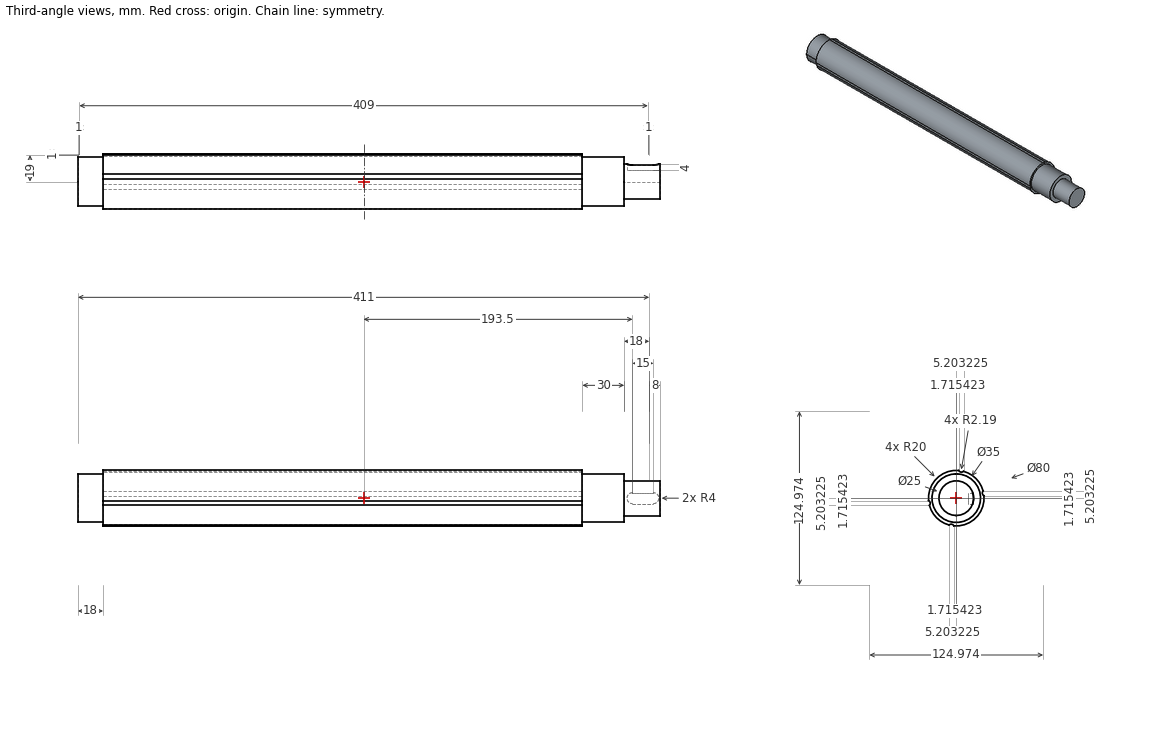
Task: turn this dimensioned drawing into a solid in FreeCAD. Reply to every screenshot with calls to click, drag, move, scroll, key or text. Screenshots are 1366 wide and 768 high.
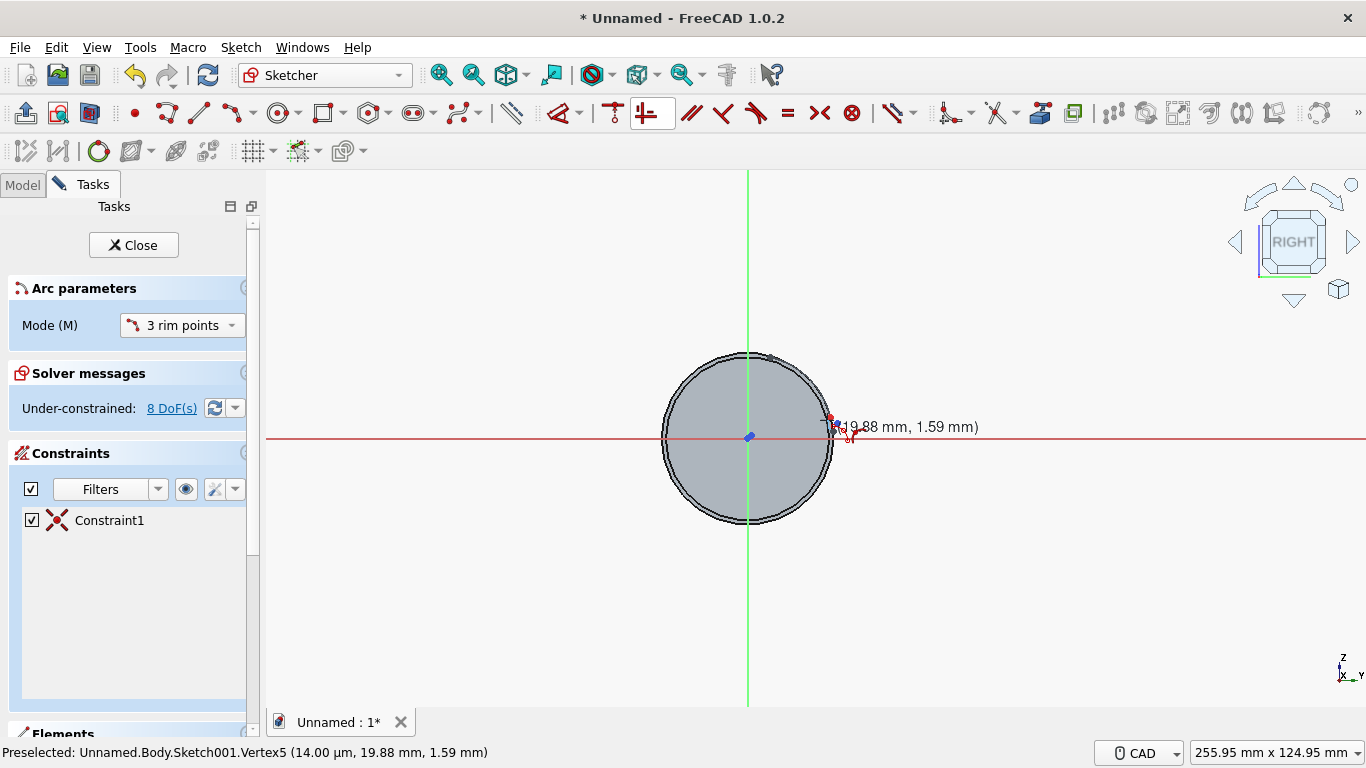
scroll(740, 524, up, 4)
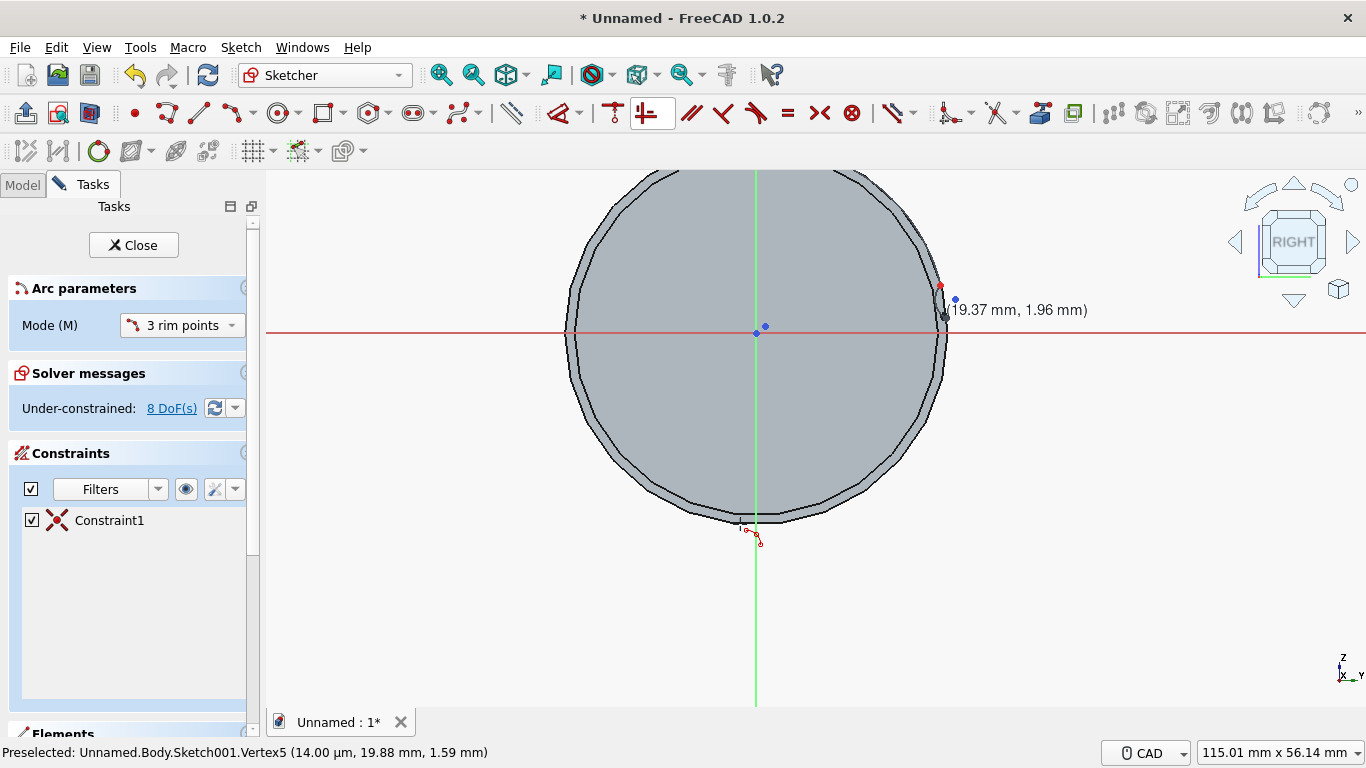
click(740, 524)
click(892, 469)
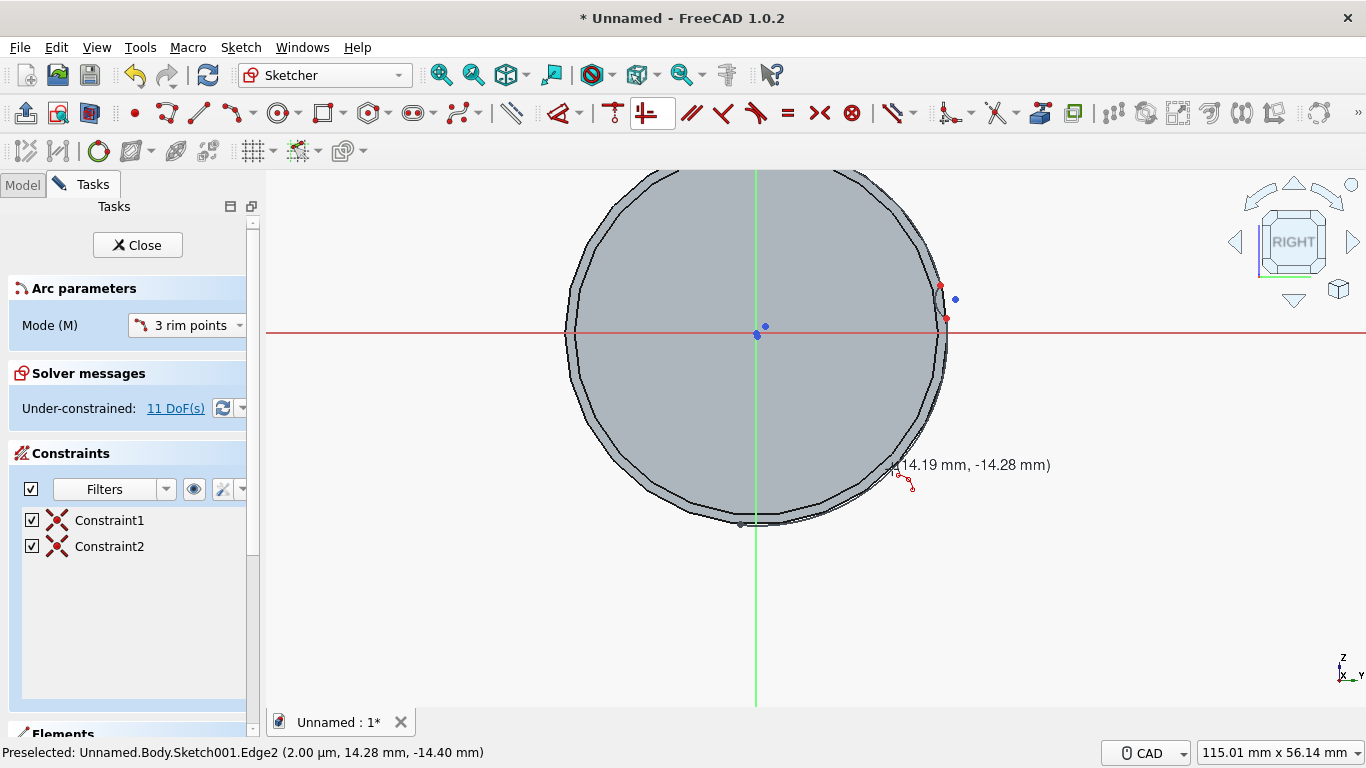
click(740, 525)
click(707, 518)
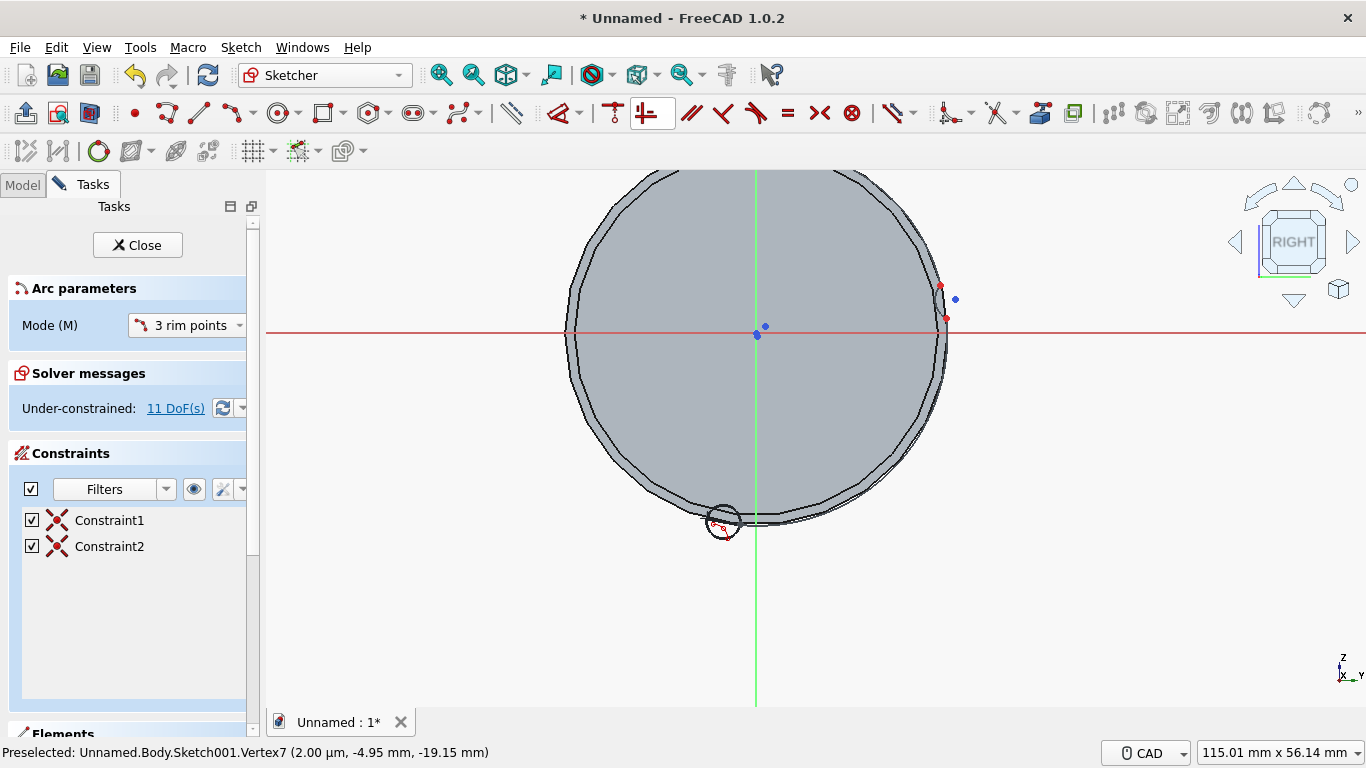
scroll(725, 513, up, 4)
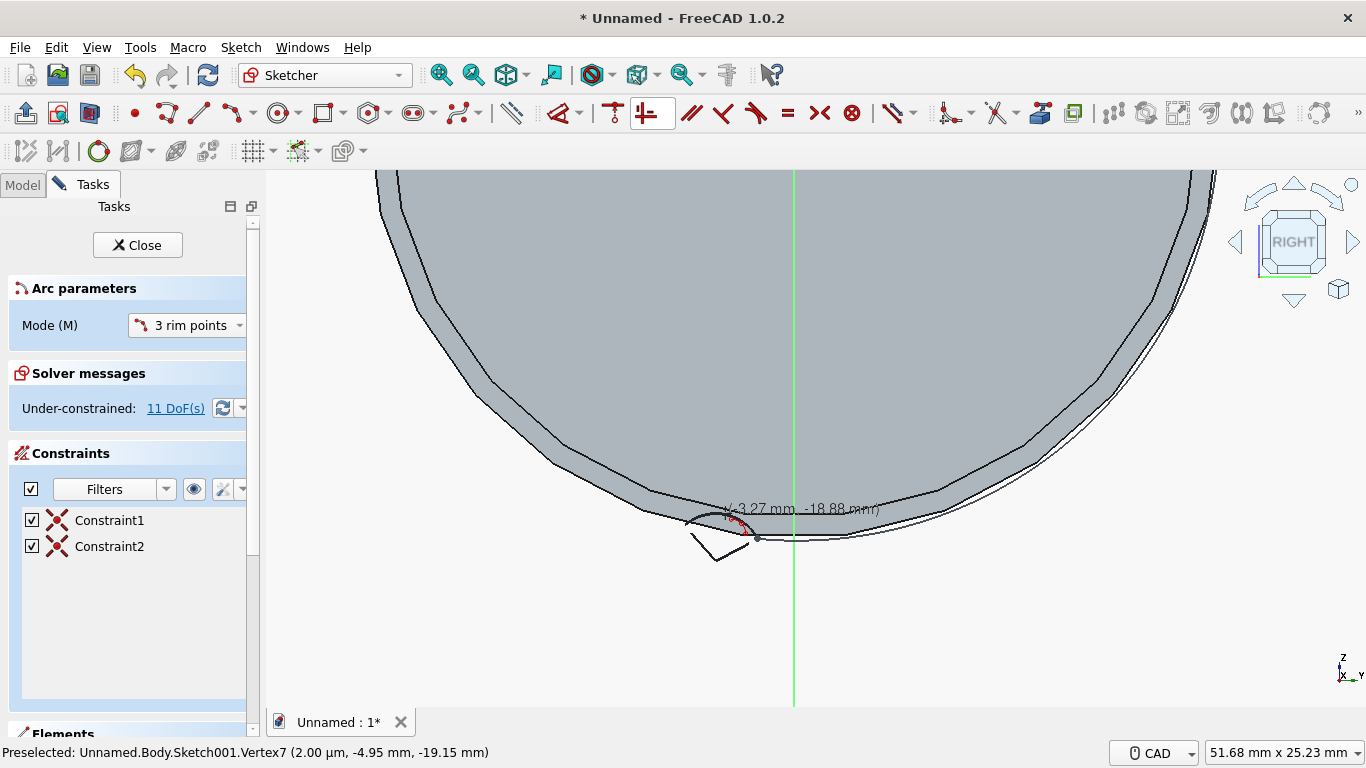
click(724, 511)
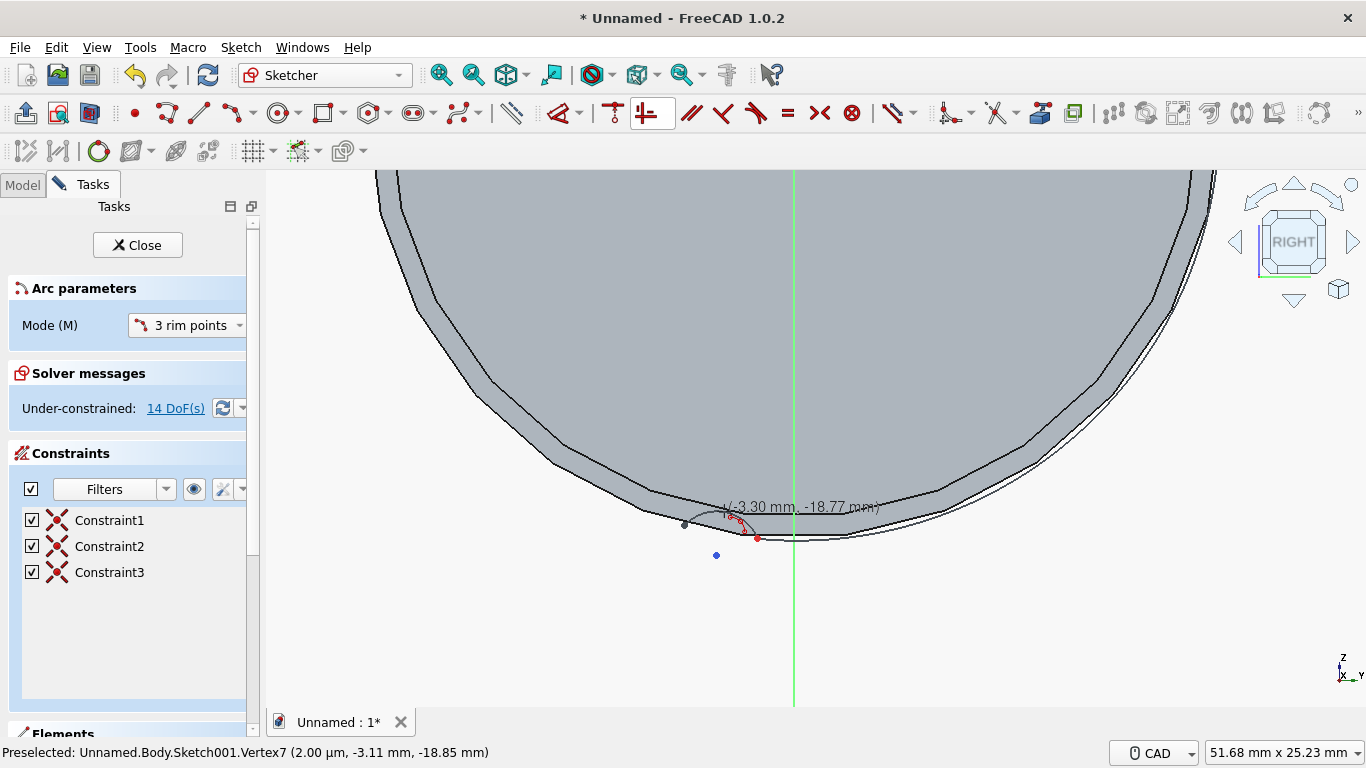
scroll(736, 521, down, 8)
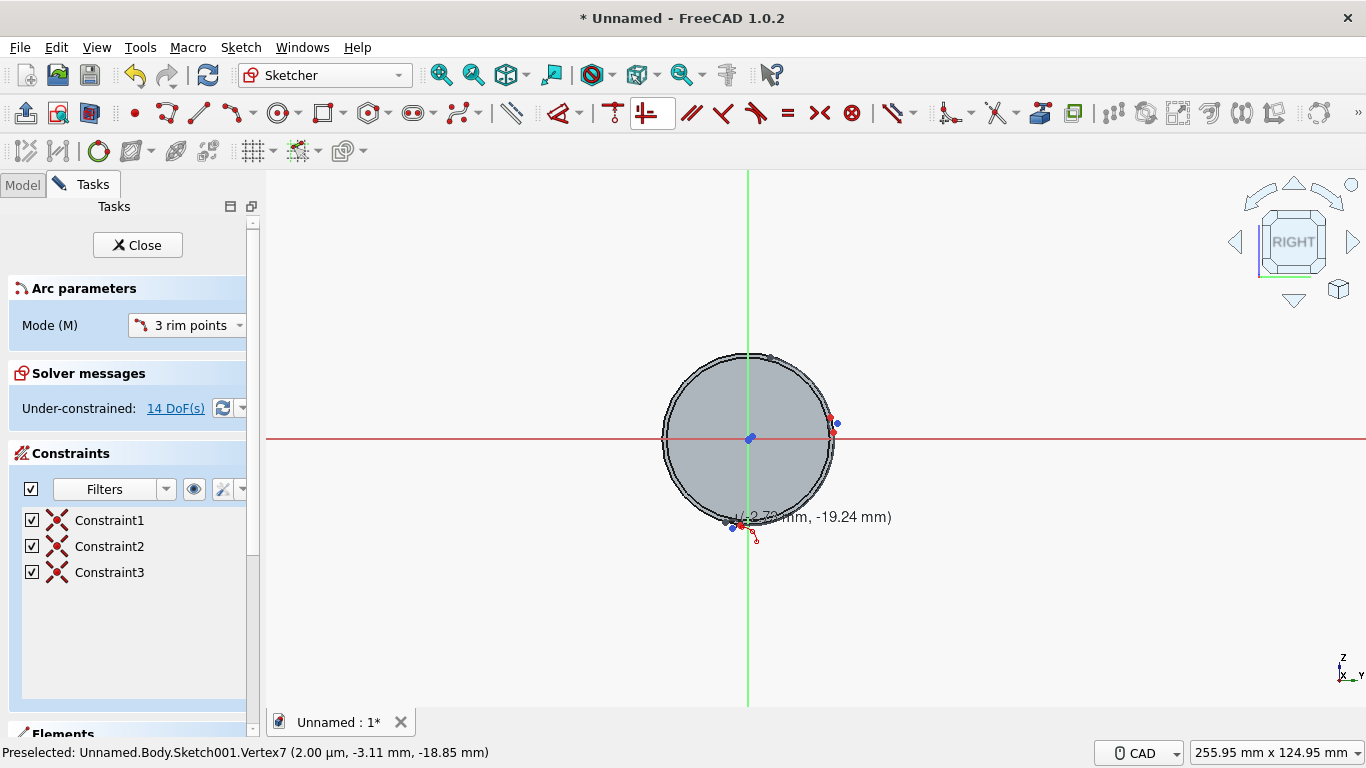
scroll(726, 522, up, 3)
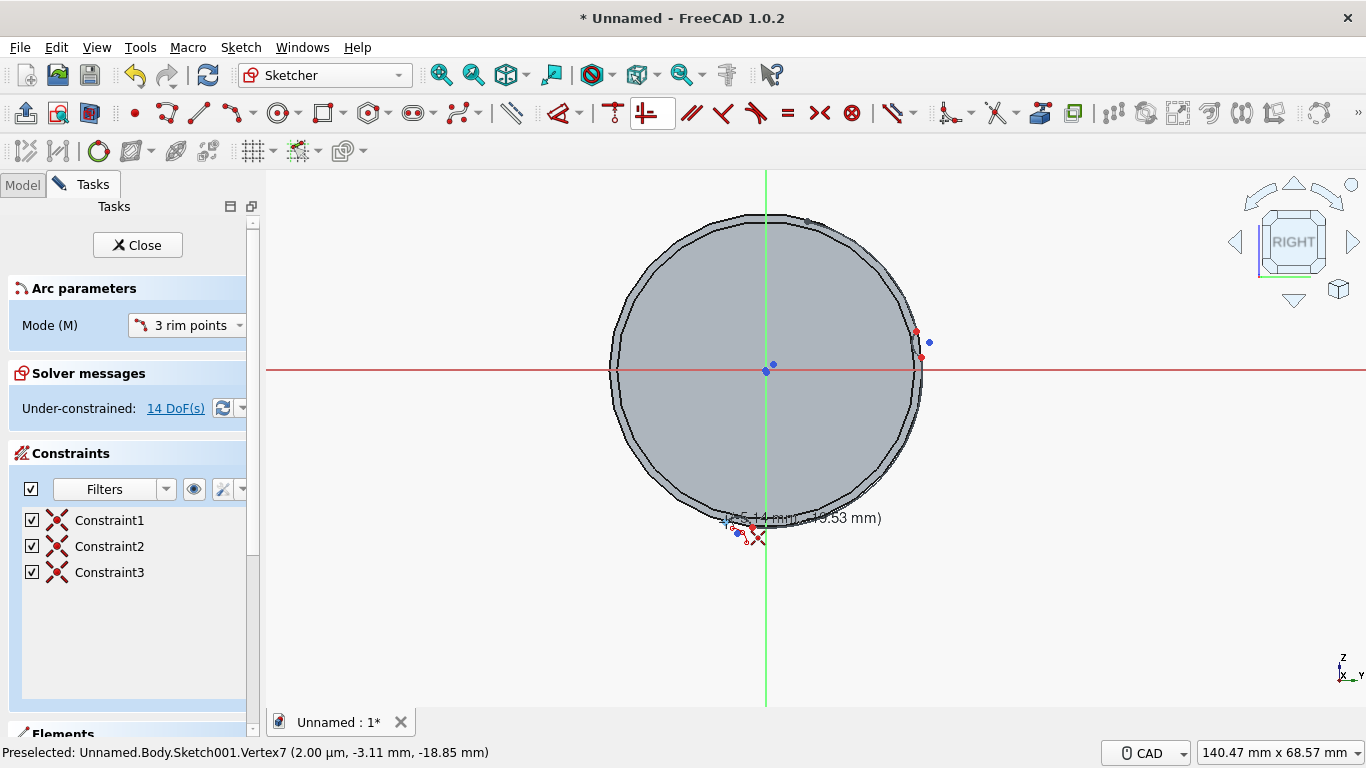
click(726, 522)
click(615, 411)
click(655, 481)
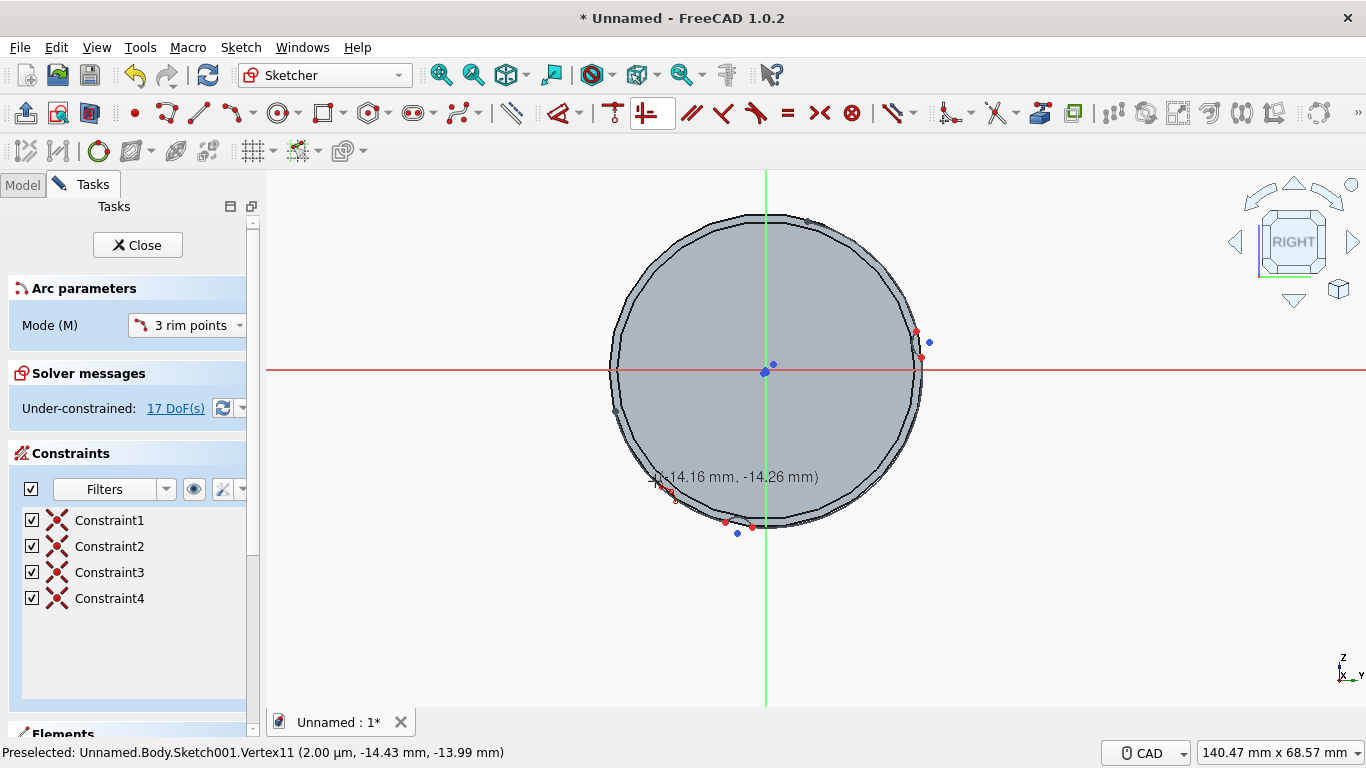
click(615, 412)
click(610, 384)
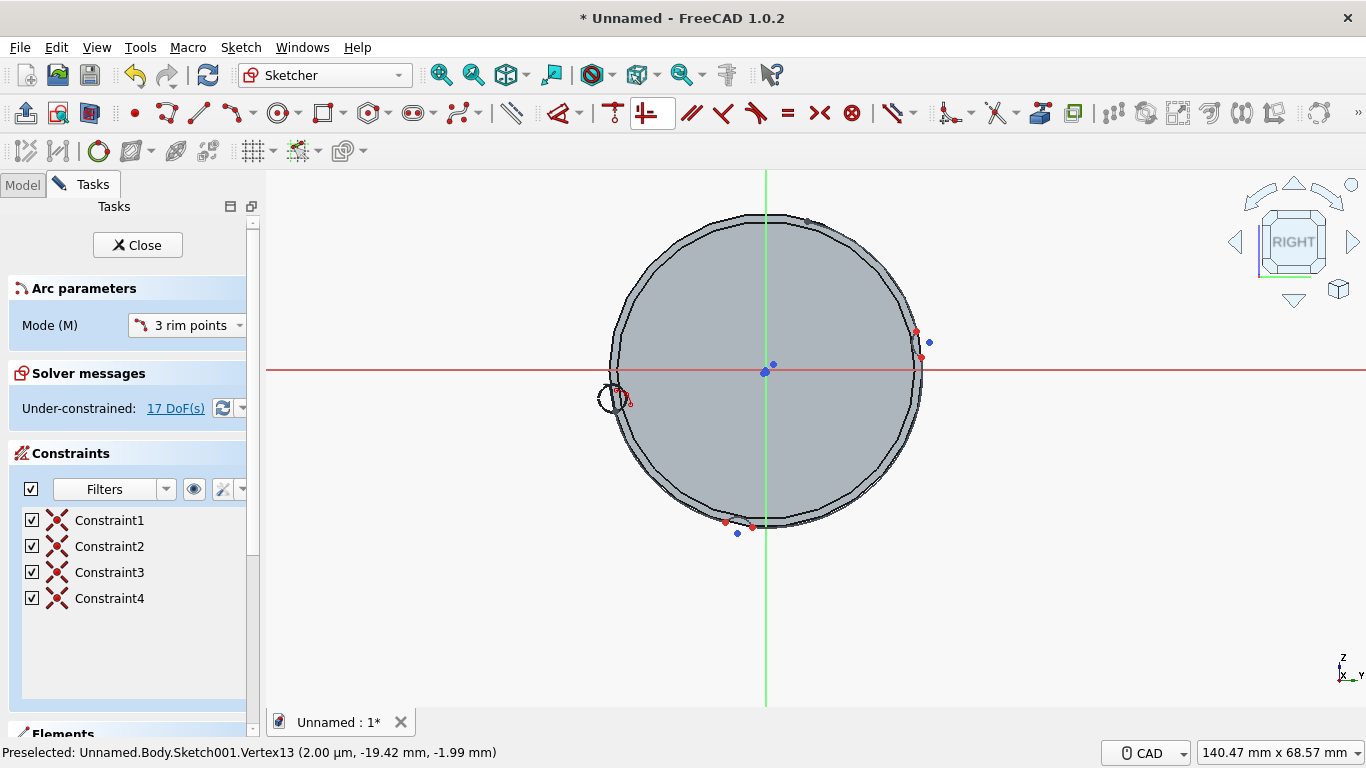
scroll(619, 396, up, 5)